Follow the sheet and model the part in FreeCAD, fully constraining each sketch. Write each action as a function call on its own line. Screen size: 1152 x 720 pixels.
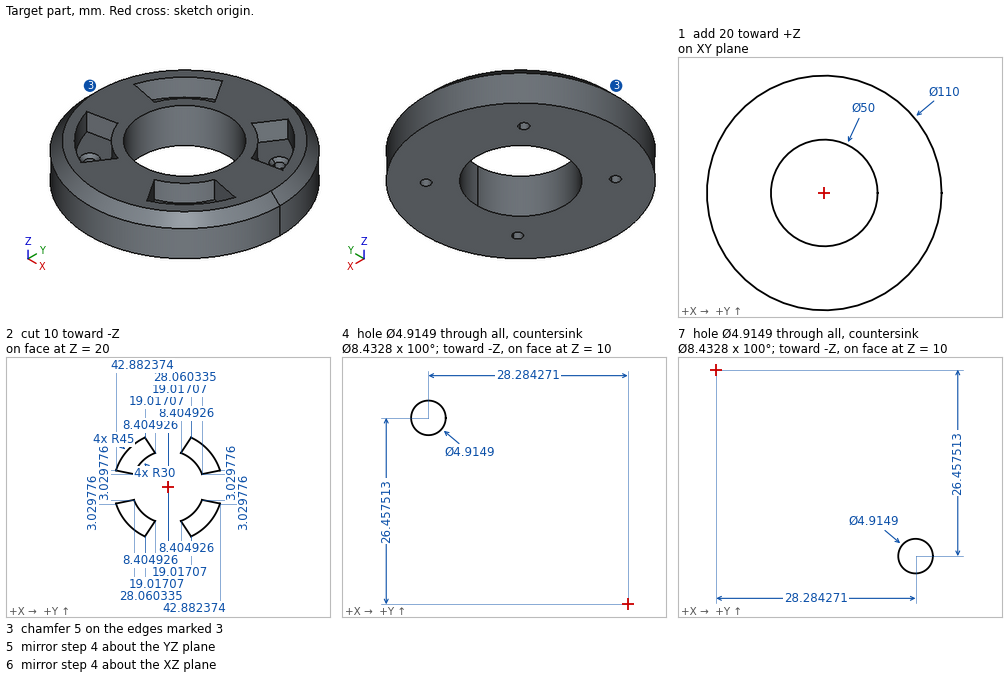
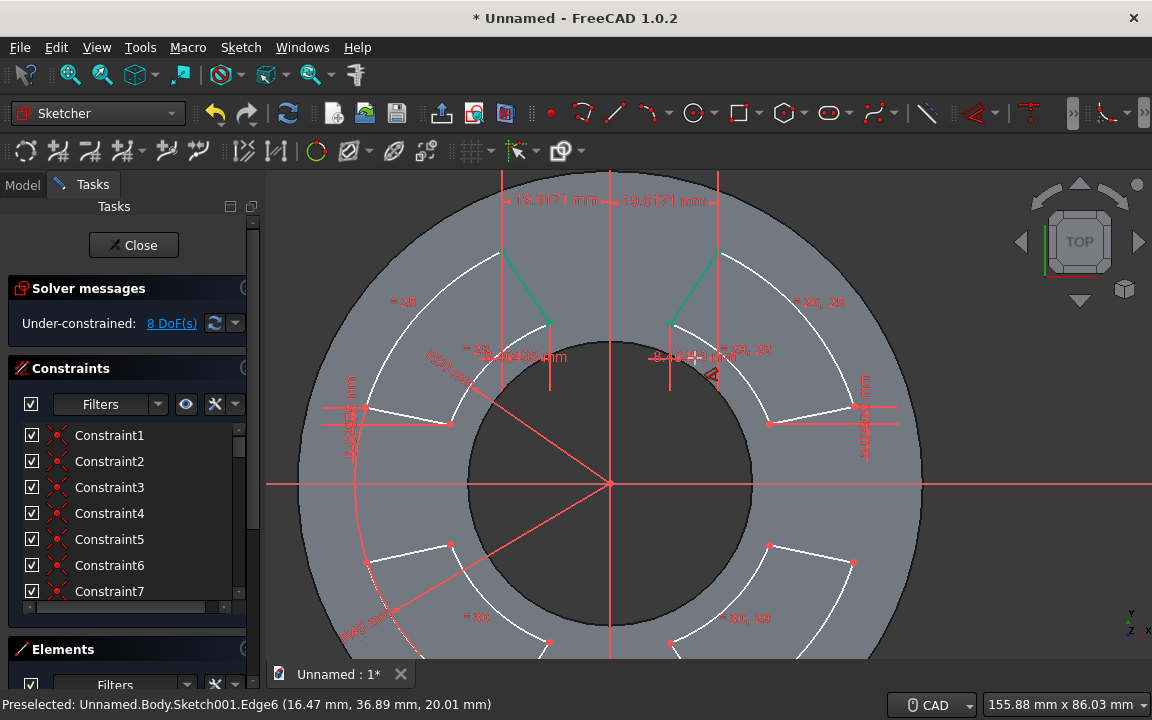
scroll(702, 274, down, 2)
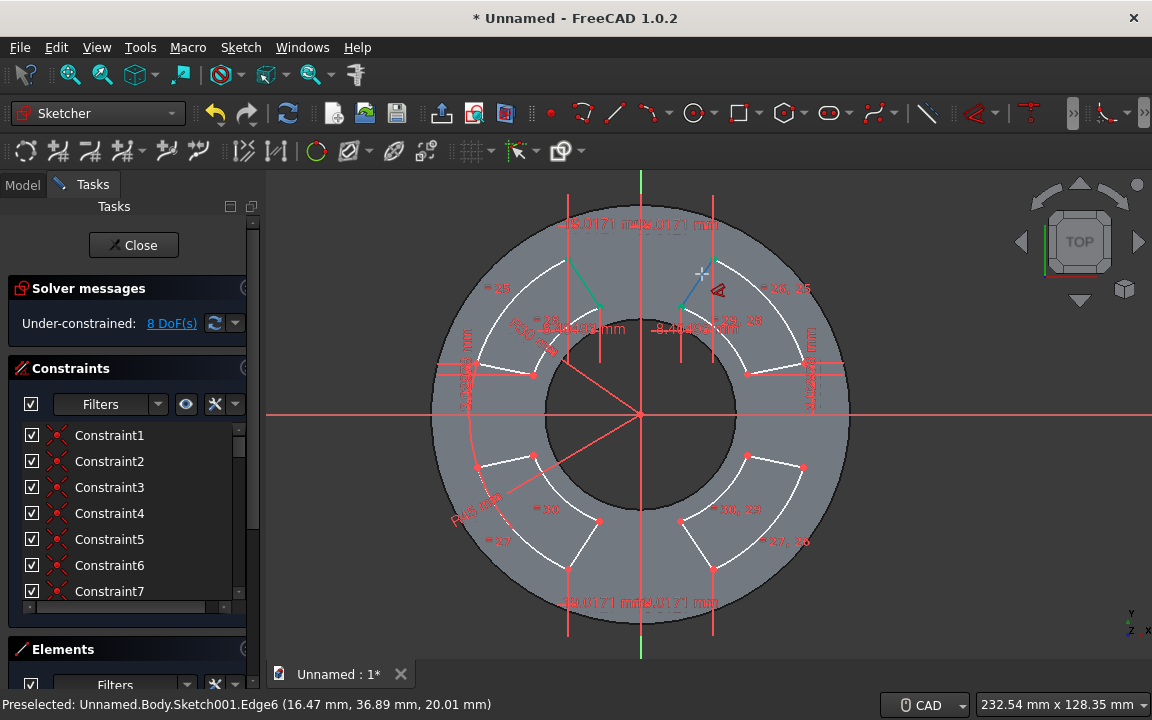
scroll(691, 536, up, 2)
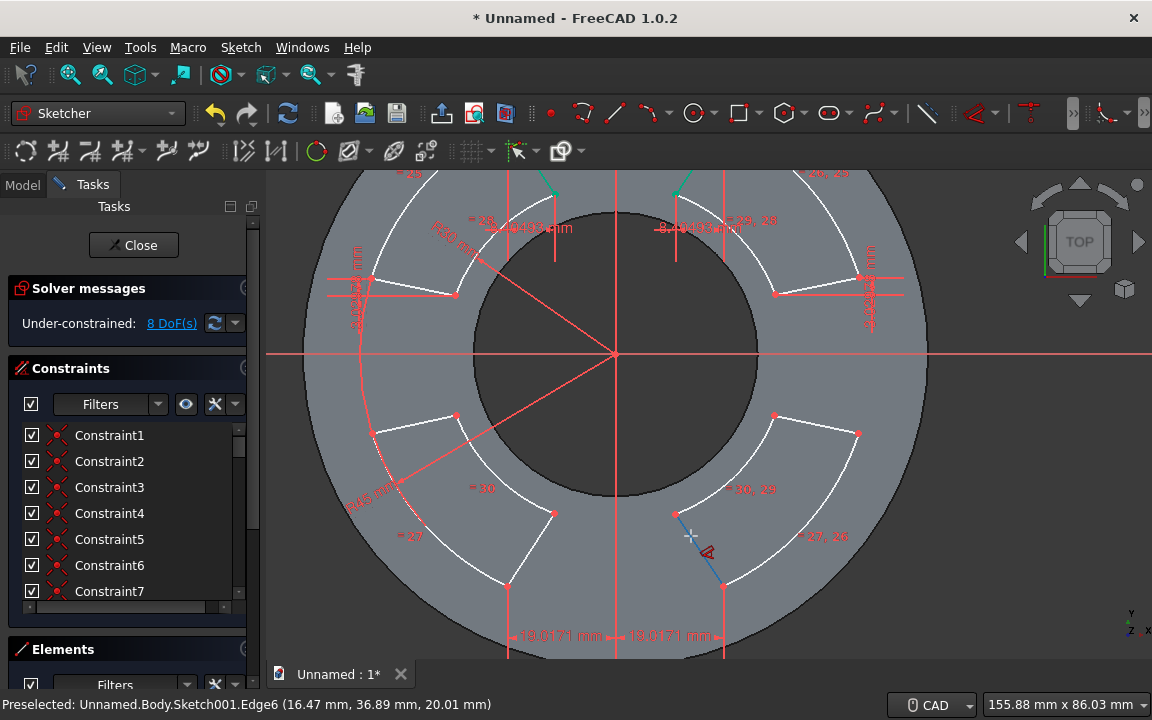
click(690, 536)
click(700, 480)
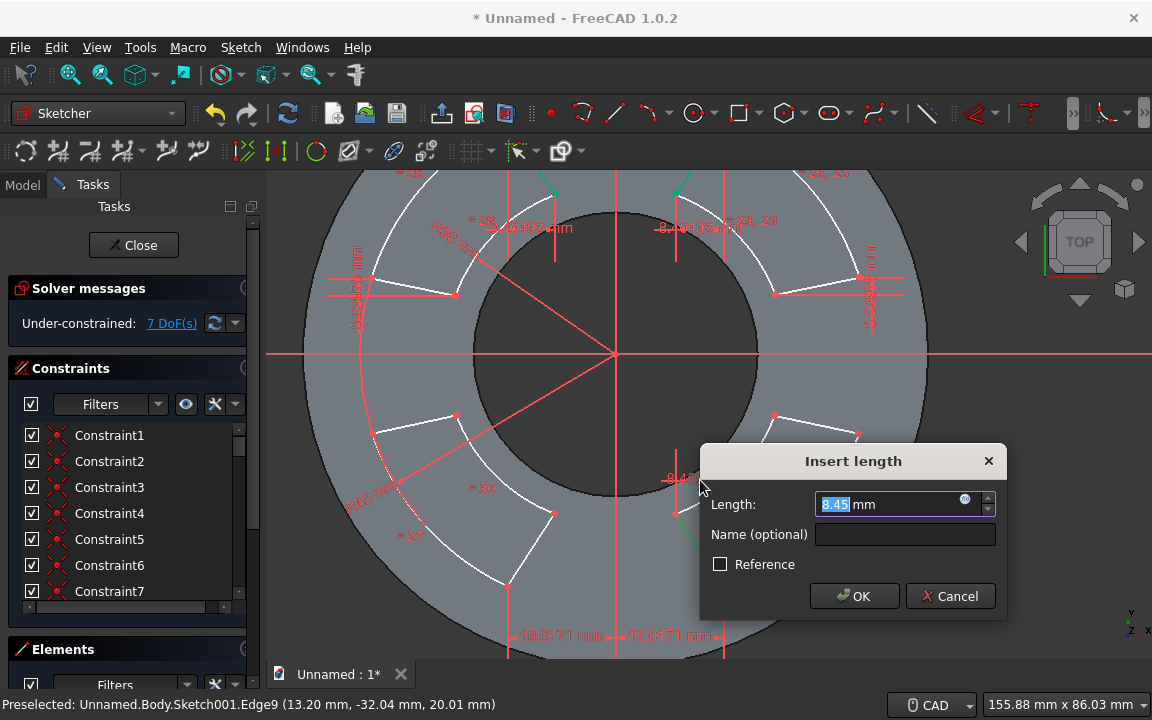
text(8.404926)
key(Return)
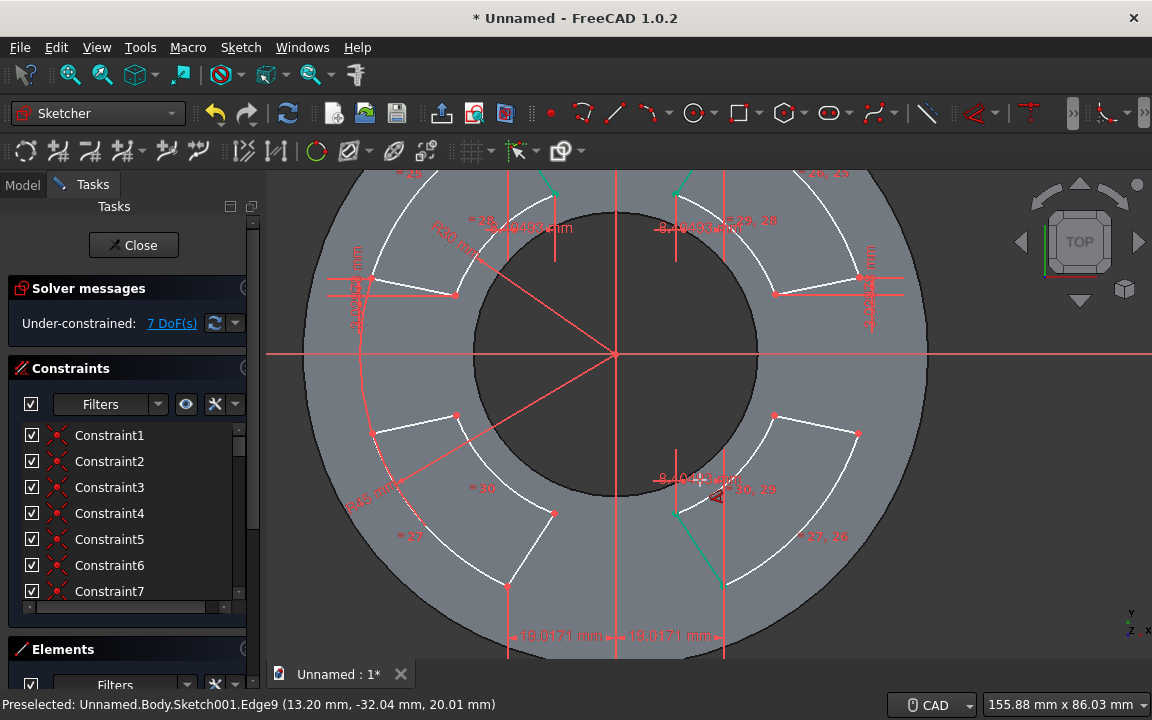
scroll(834, 428, up, 5)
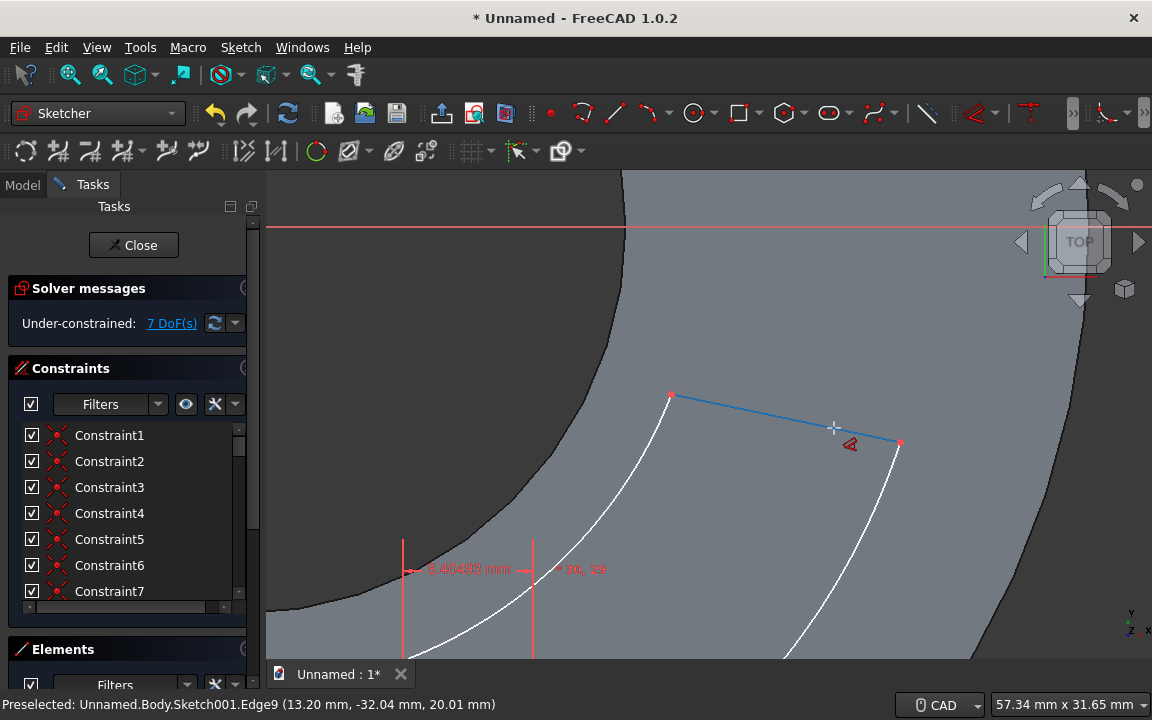
click(832, 428)
click(934, 418)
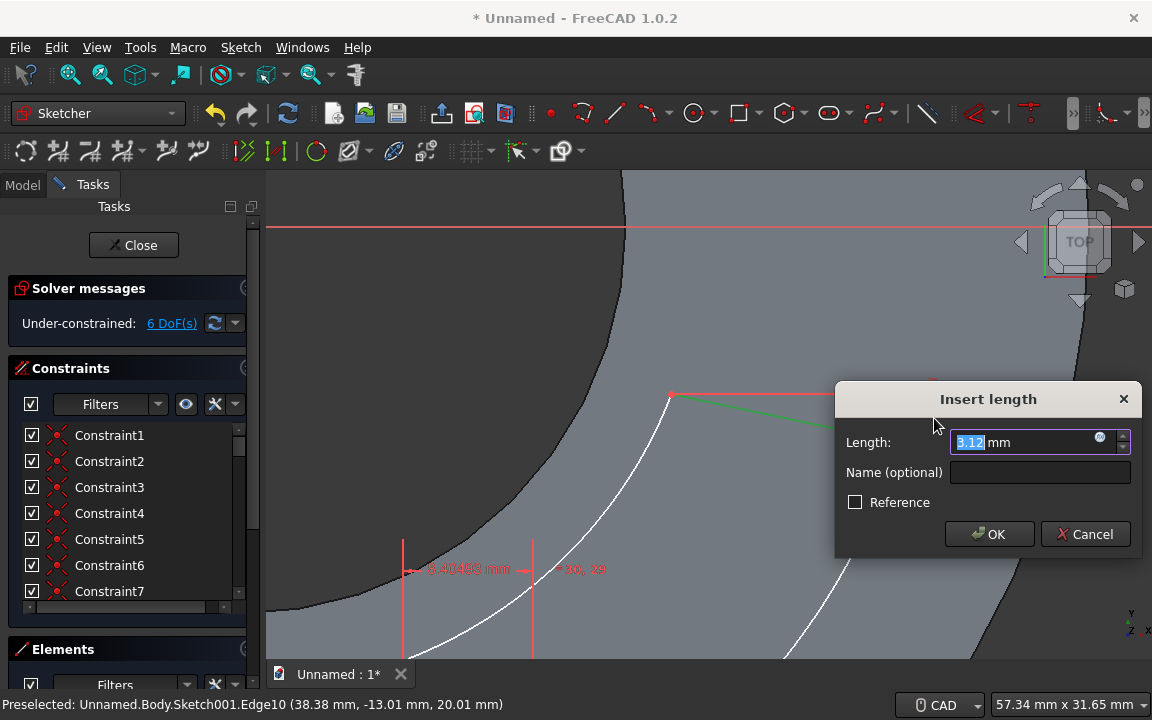
text(3.029776)
key(Return)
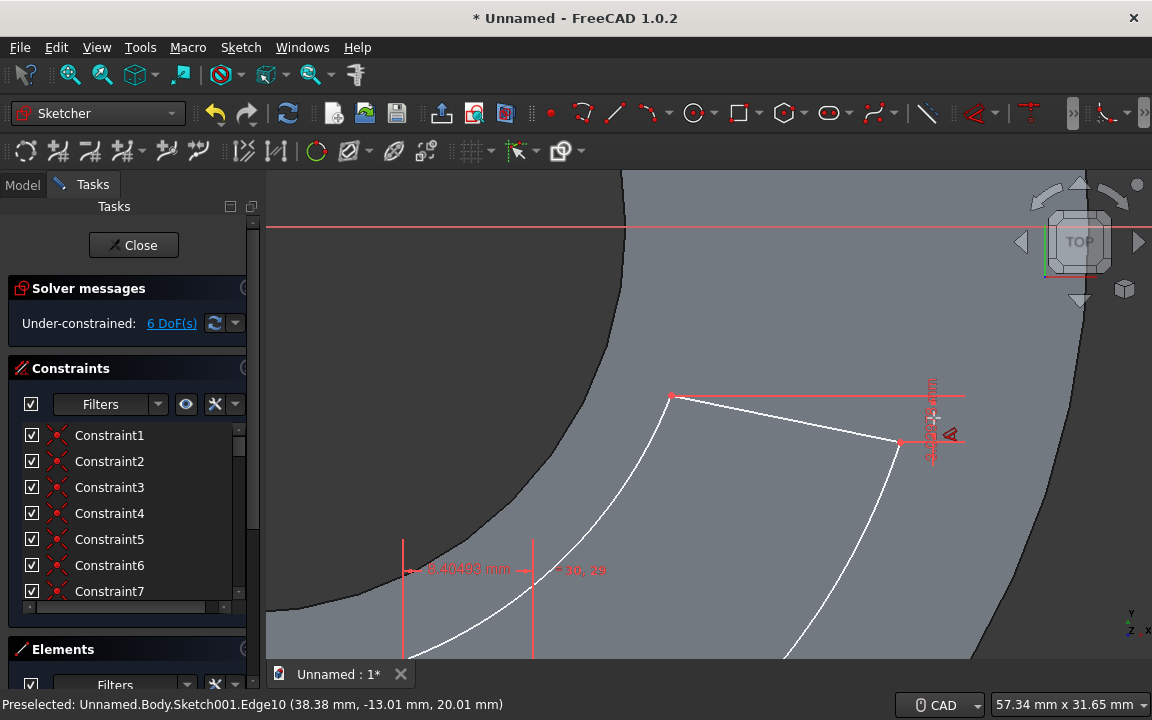
scroll(772, 476, down, 7)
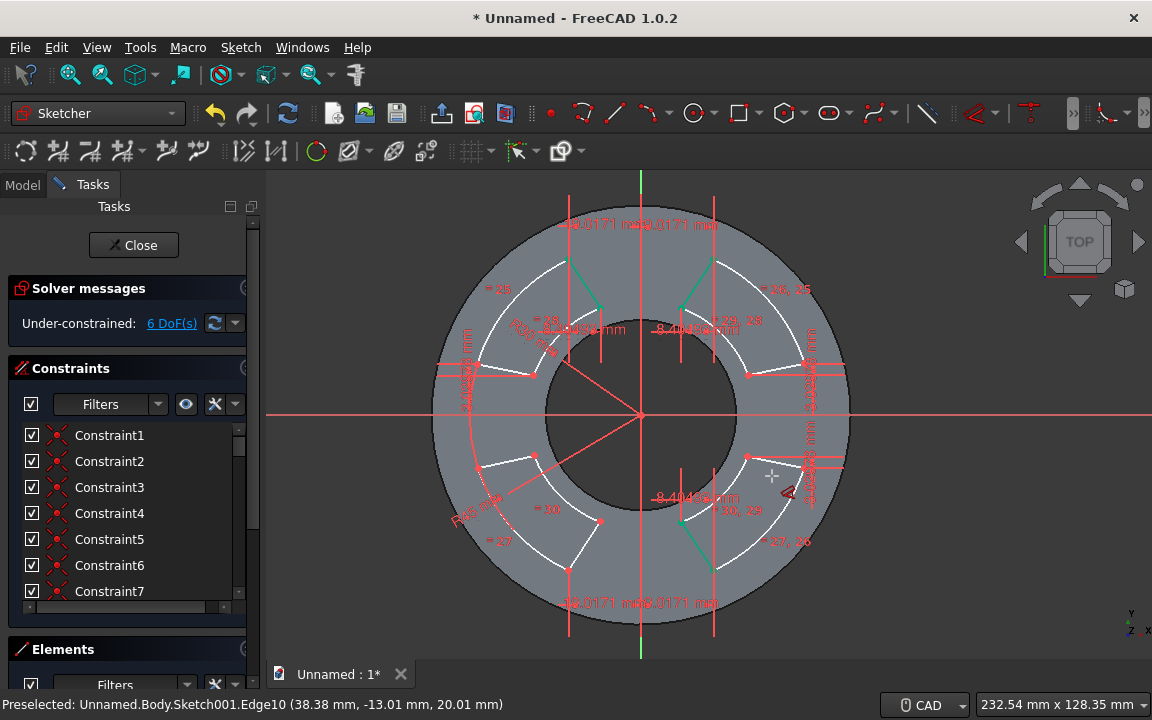
scroll(517, 460, up, 7)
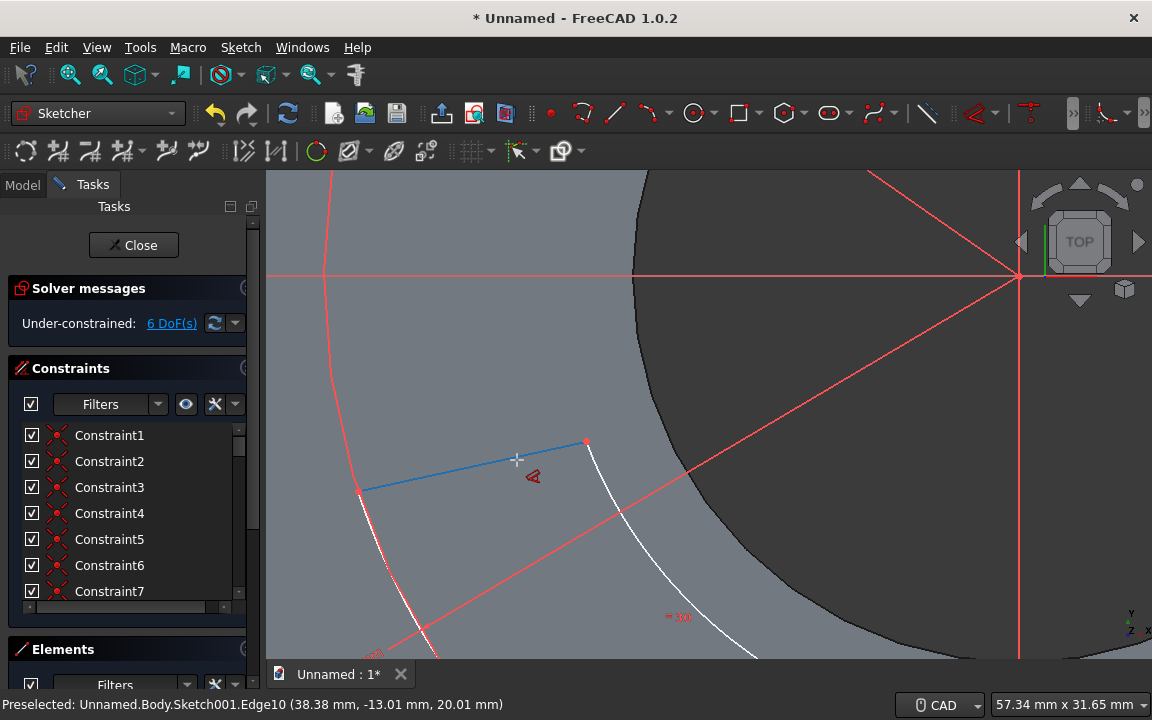
click(518, 457)
click(324, 467)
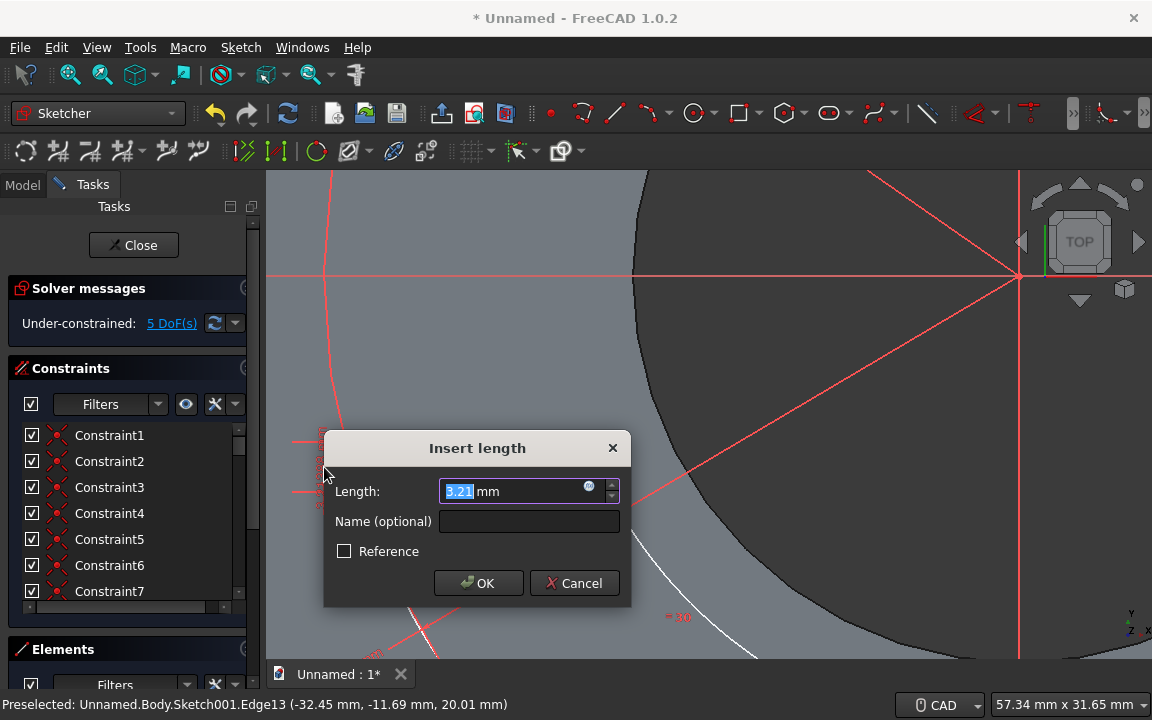
text(3.029776)
key(Return)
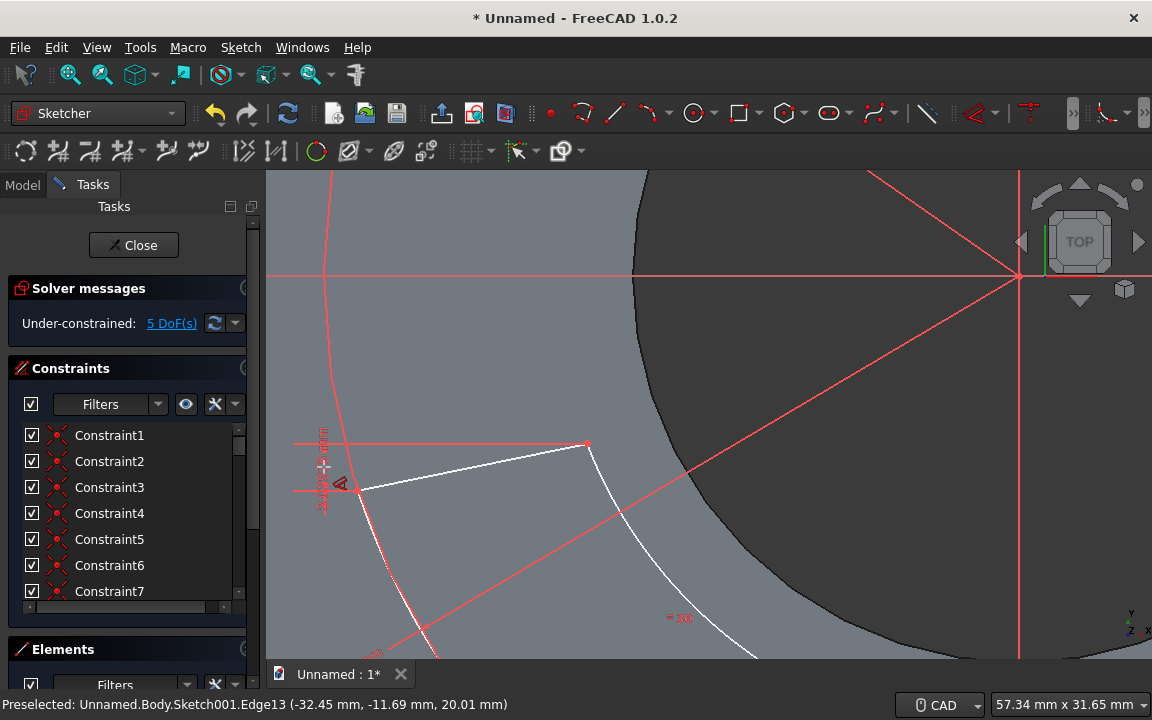
scroll(517, 460, down, 7)